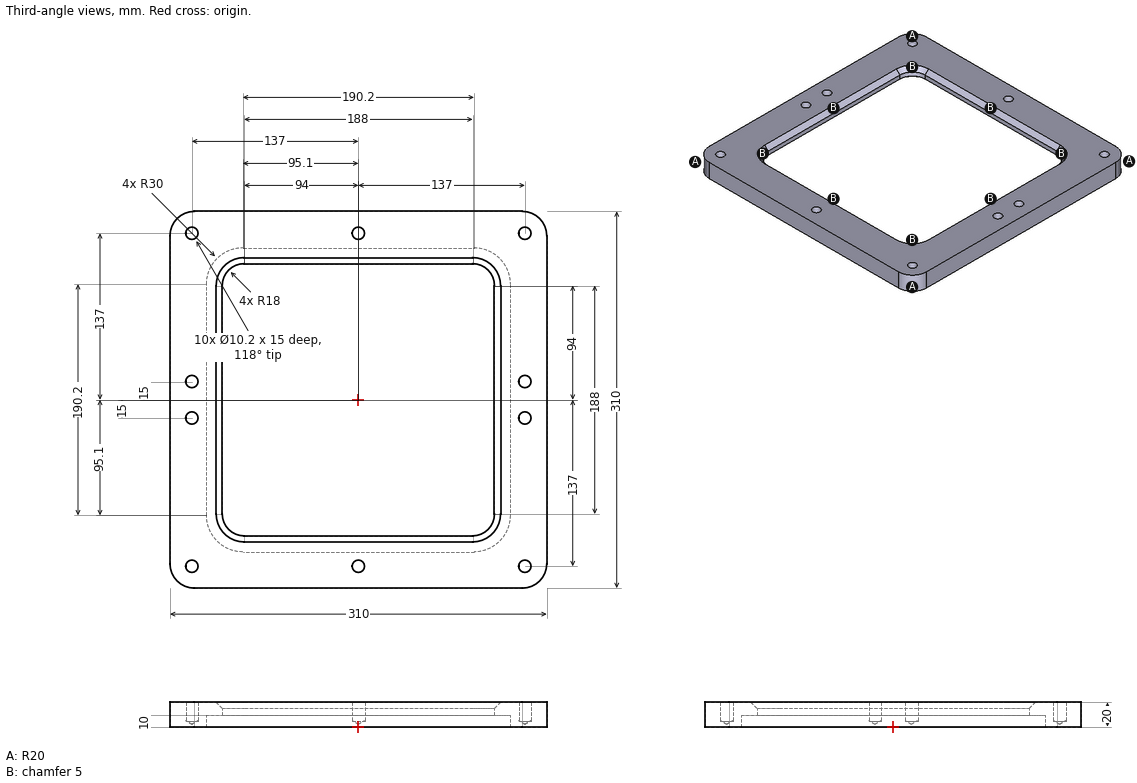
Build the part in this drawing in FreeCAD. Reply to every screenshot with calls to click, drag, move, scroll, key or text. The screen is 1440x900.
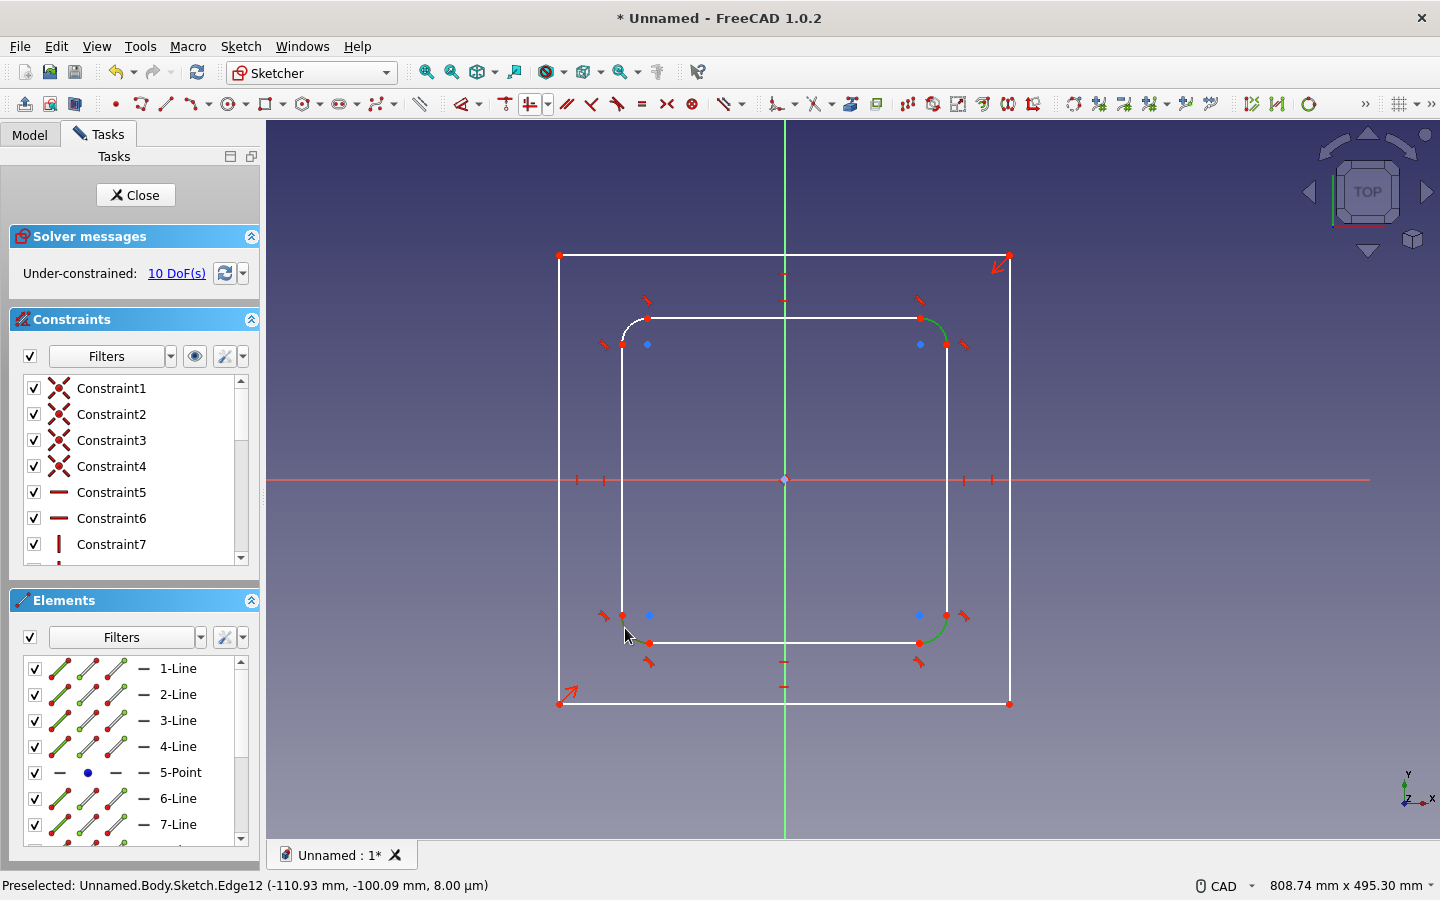
click(636, 321)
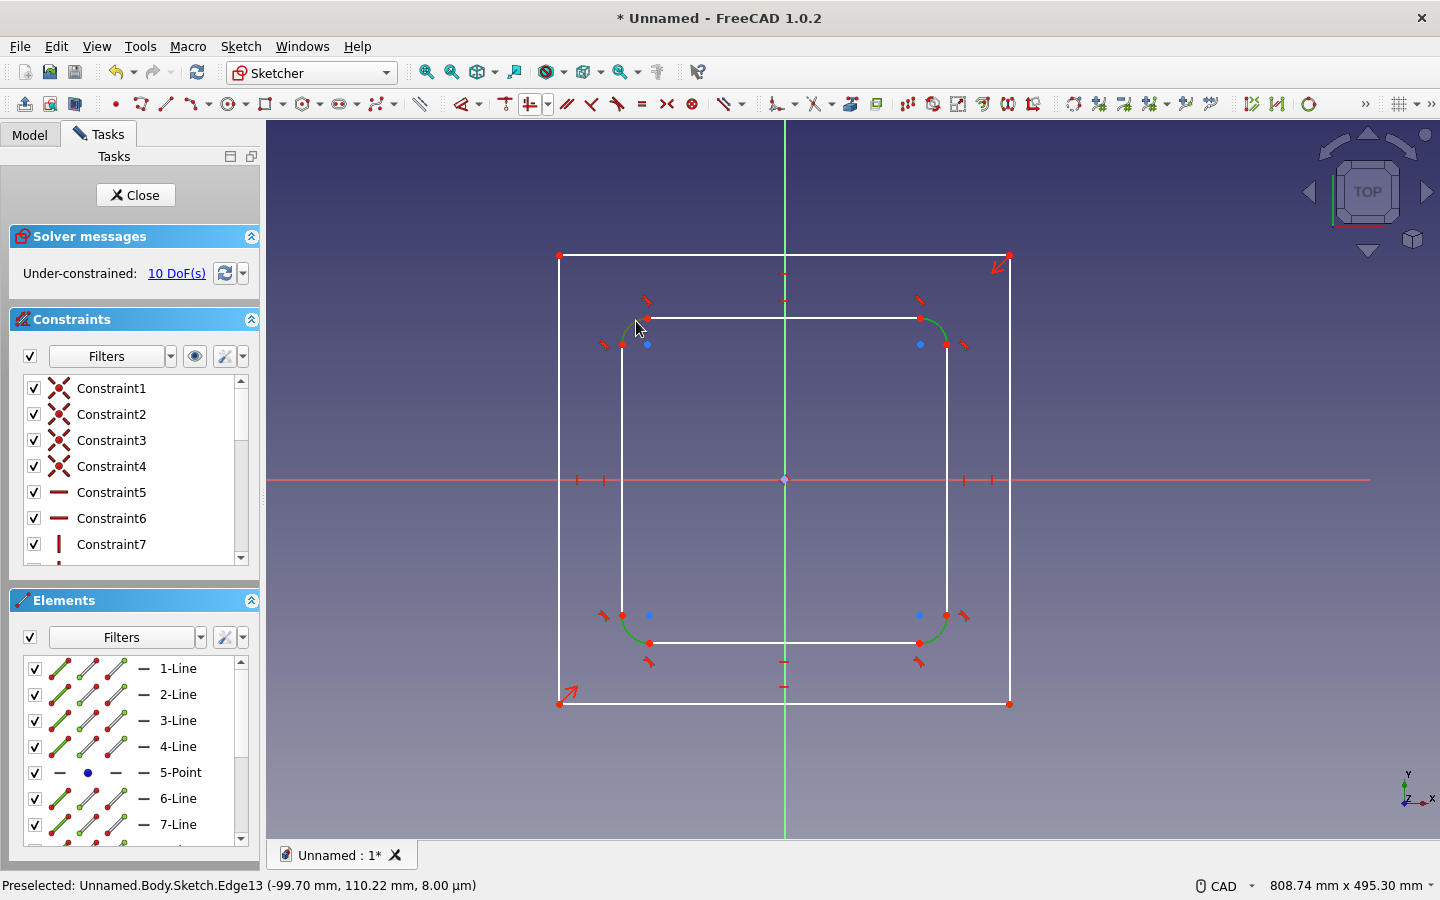
click(642, 104)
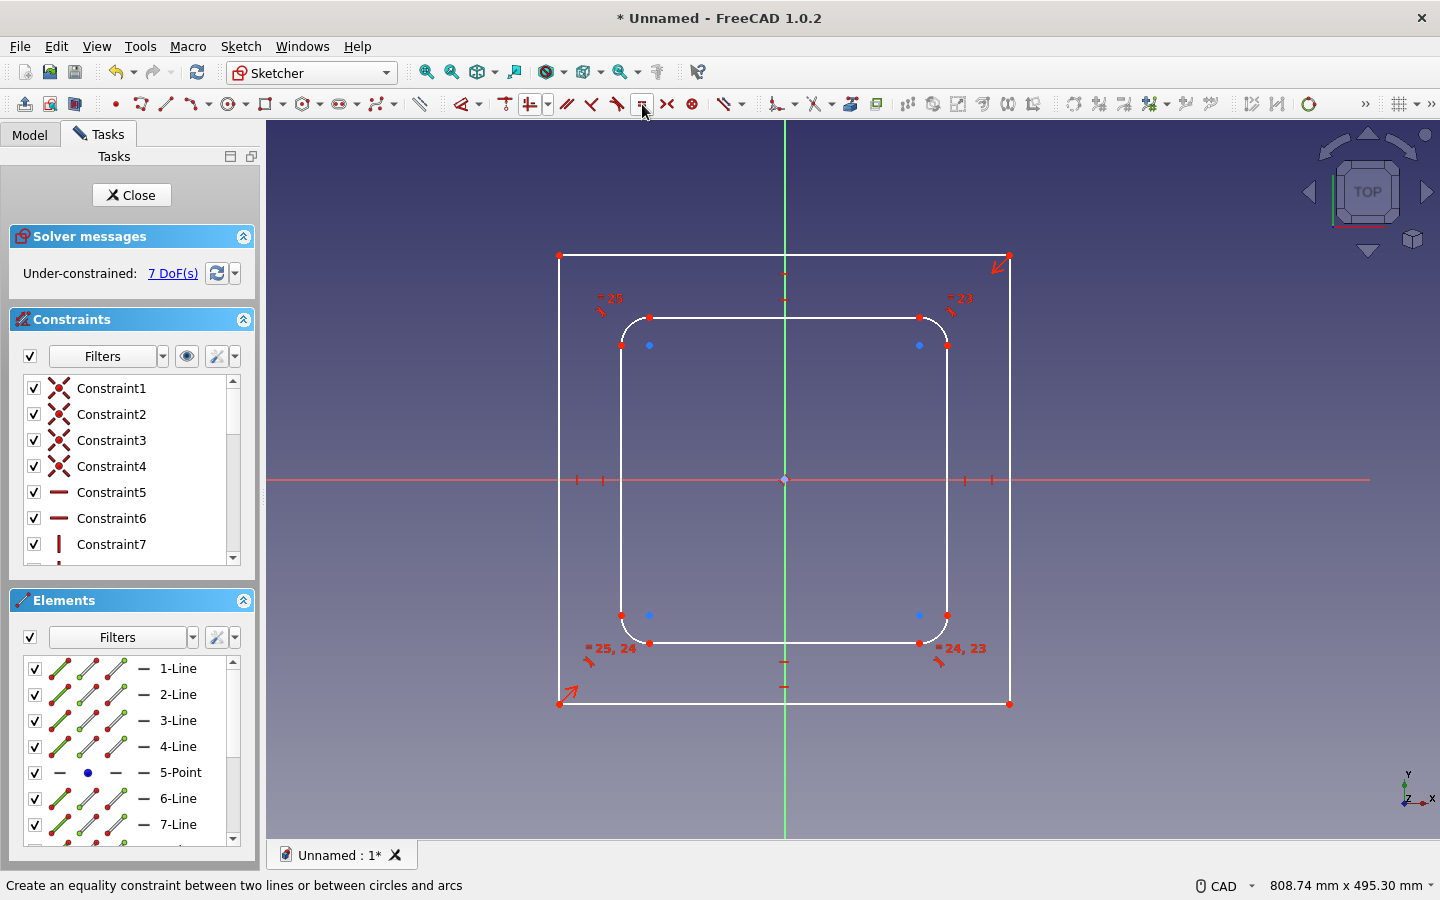
scroll(944, 333, up, 3)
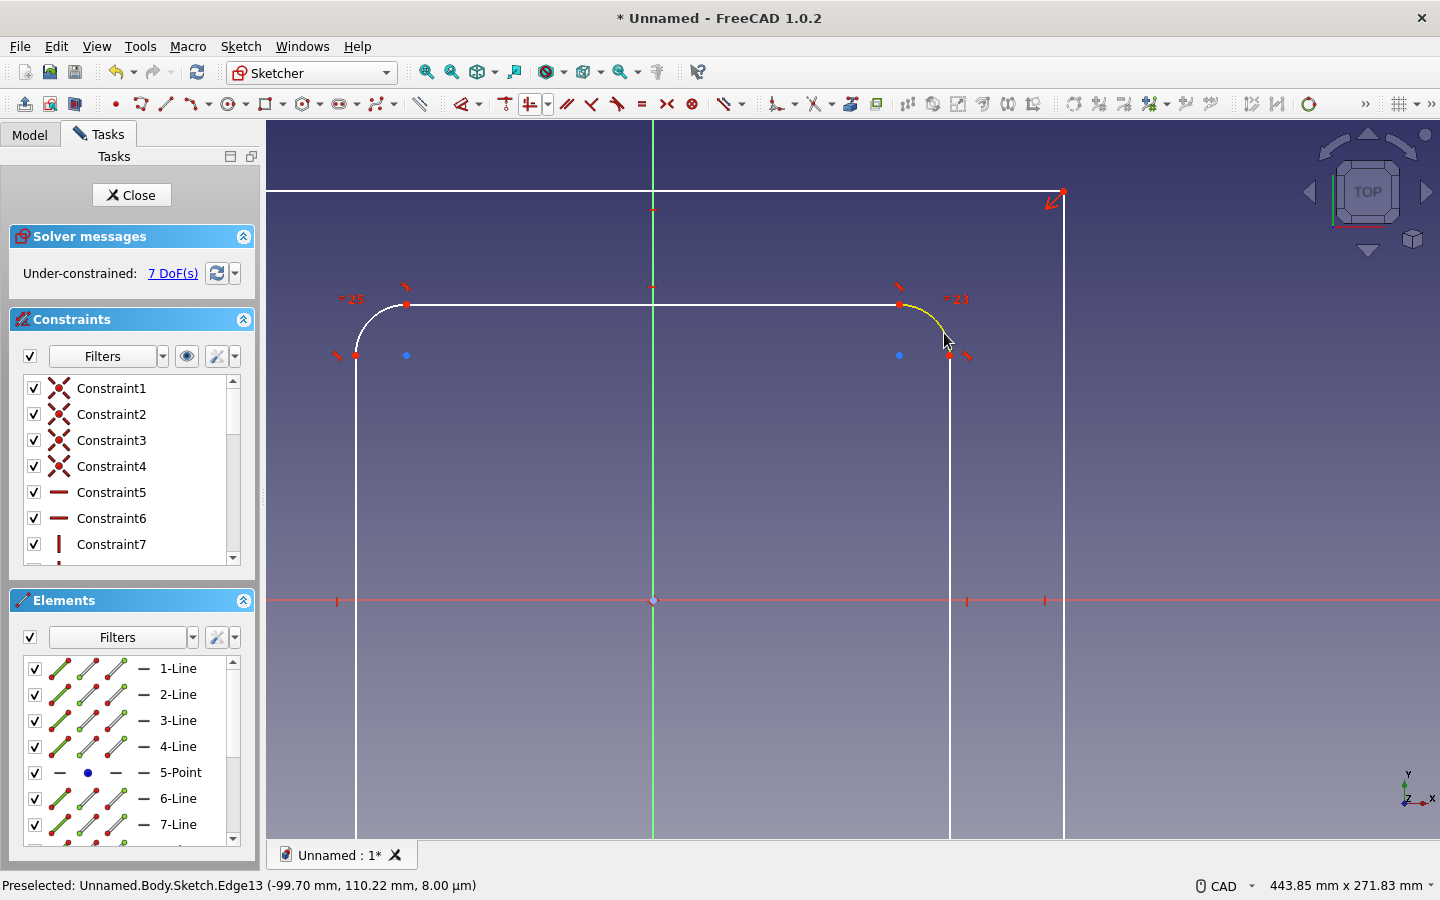
click(944, 332)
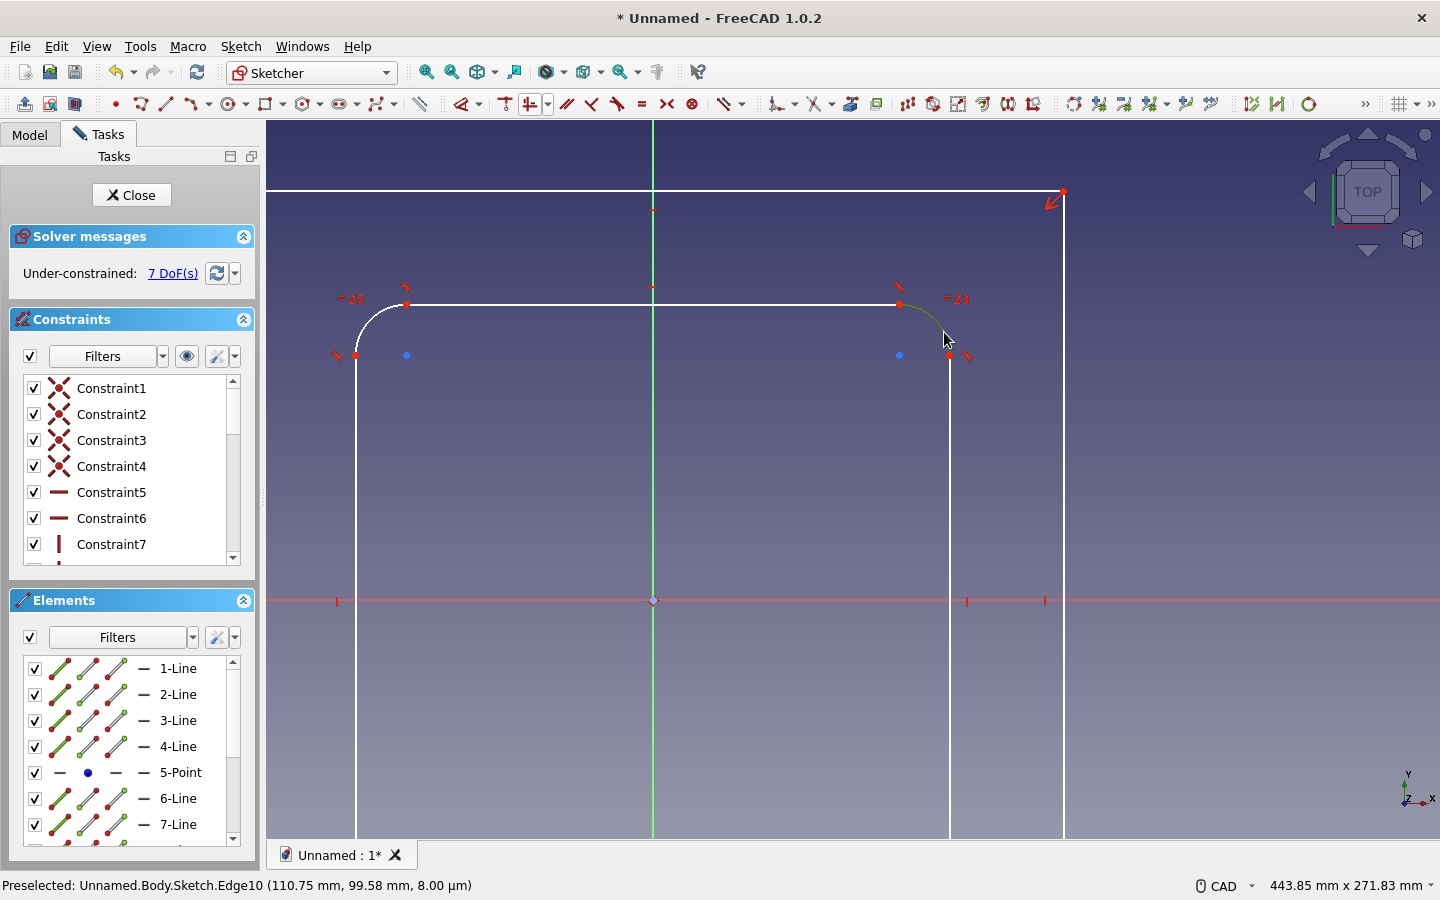
key(k)
key(r)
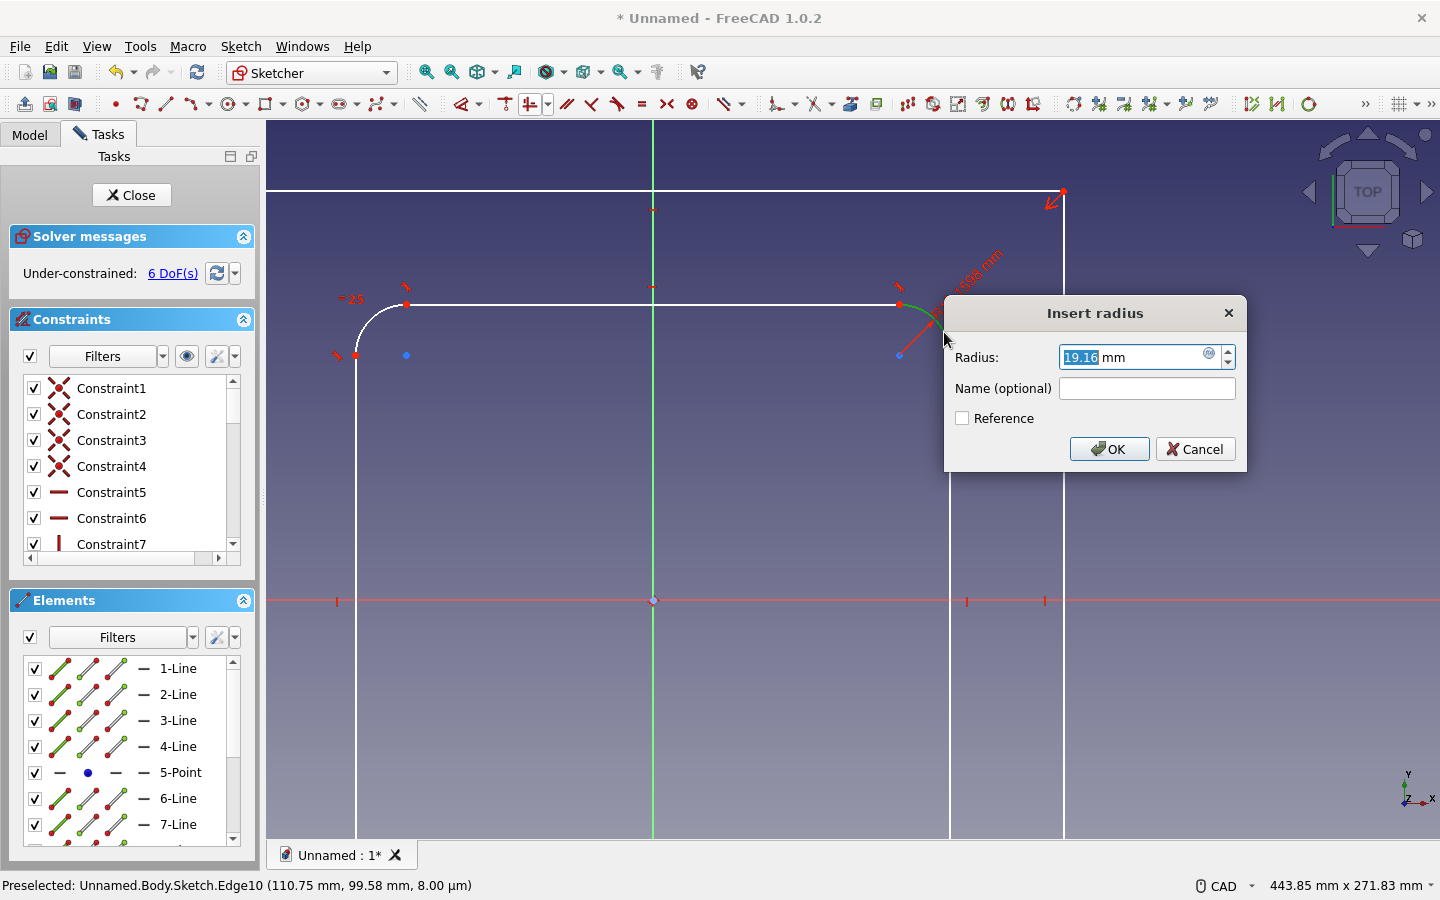
text(18)
key(Return)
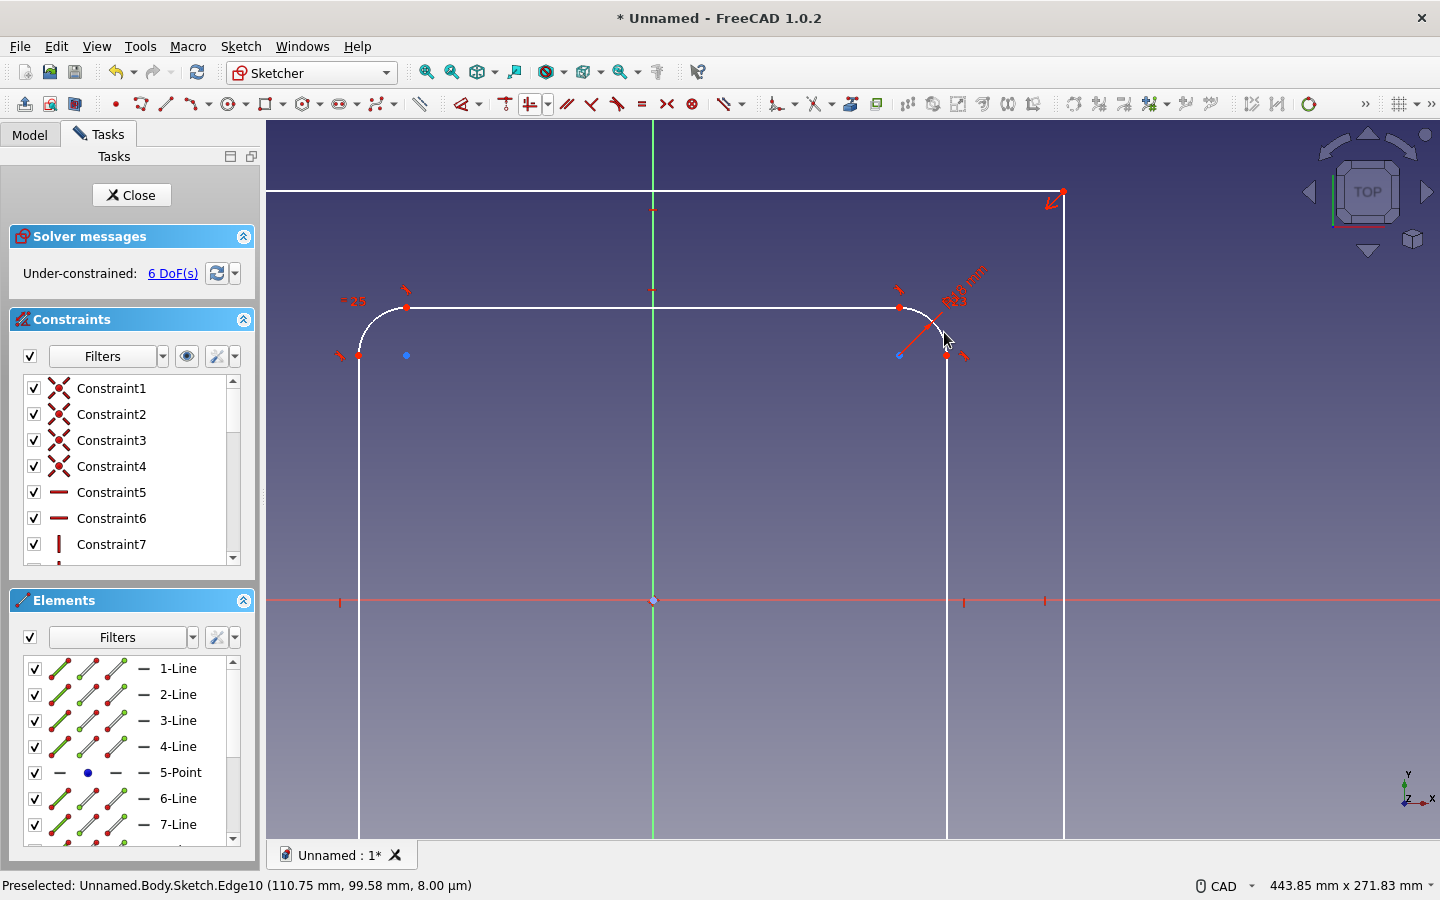
scroll(944, 333, down, 3)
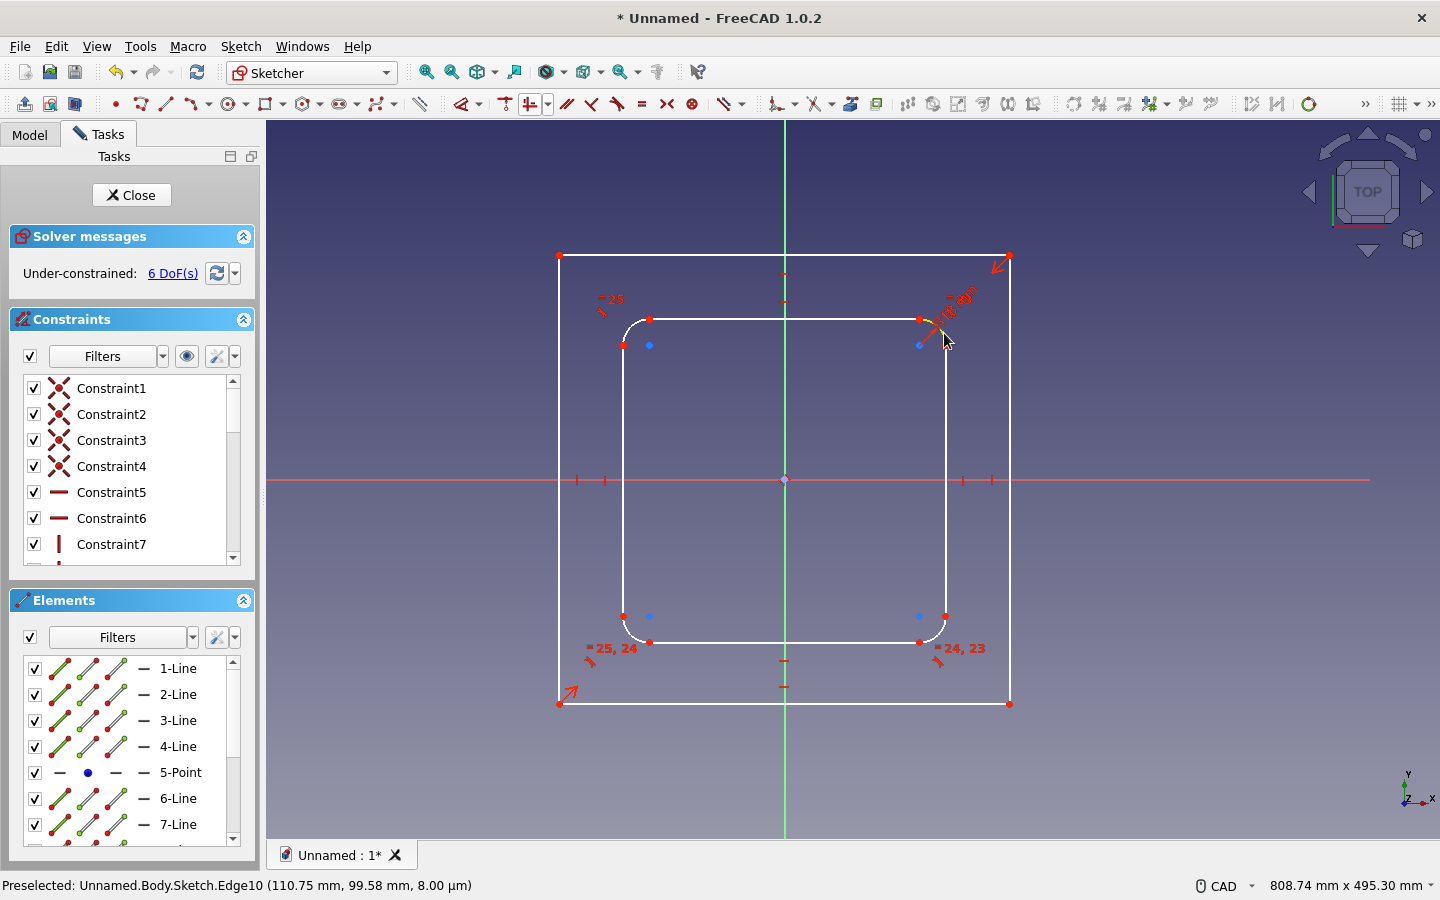
click(695, 704)